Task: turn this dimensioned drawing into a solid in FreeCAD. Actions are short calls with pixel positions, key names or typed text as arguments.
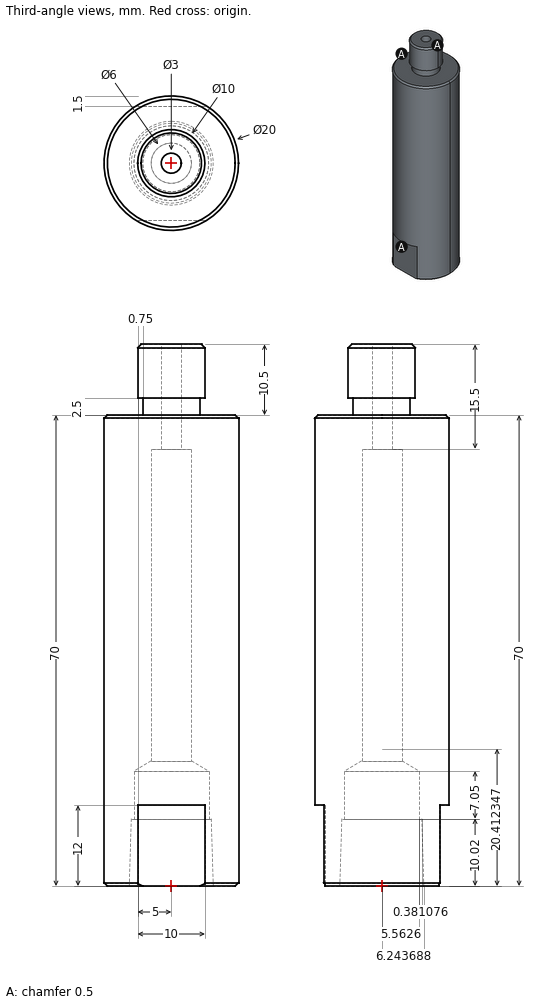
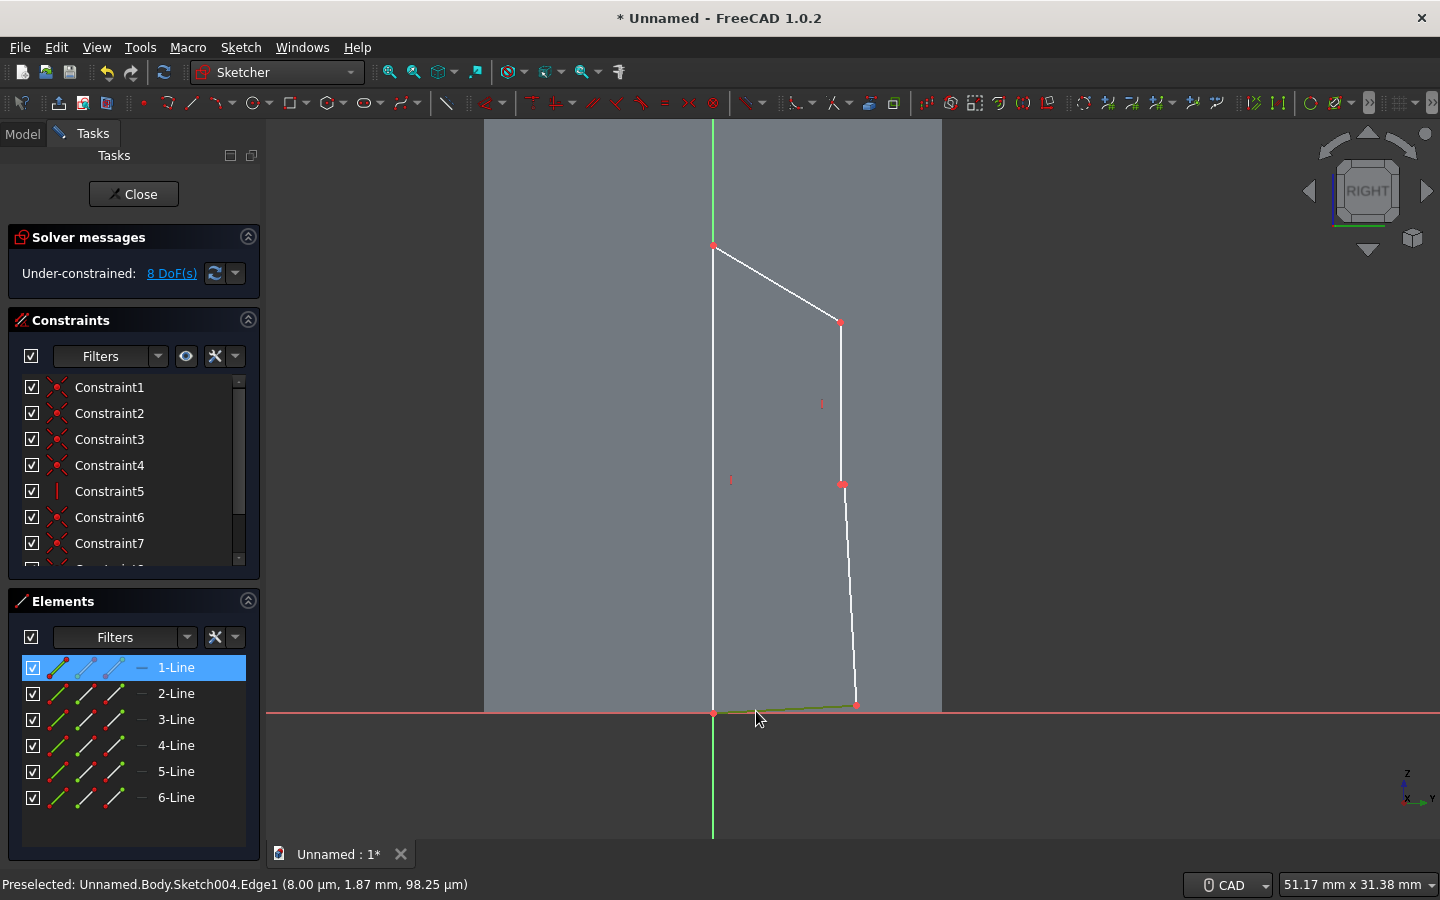
click(574, 104)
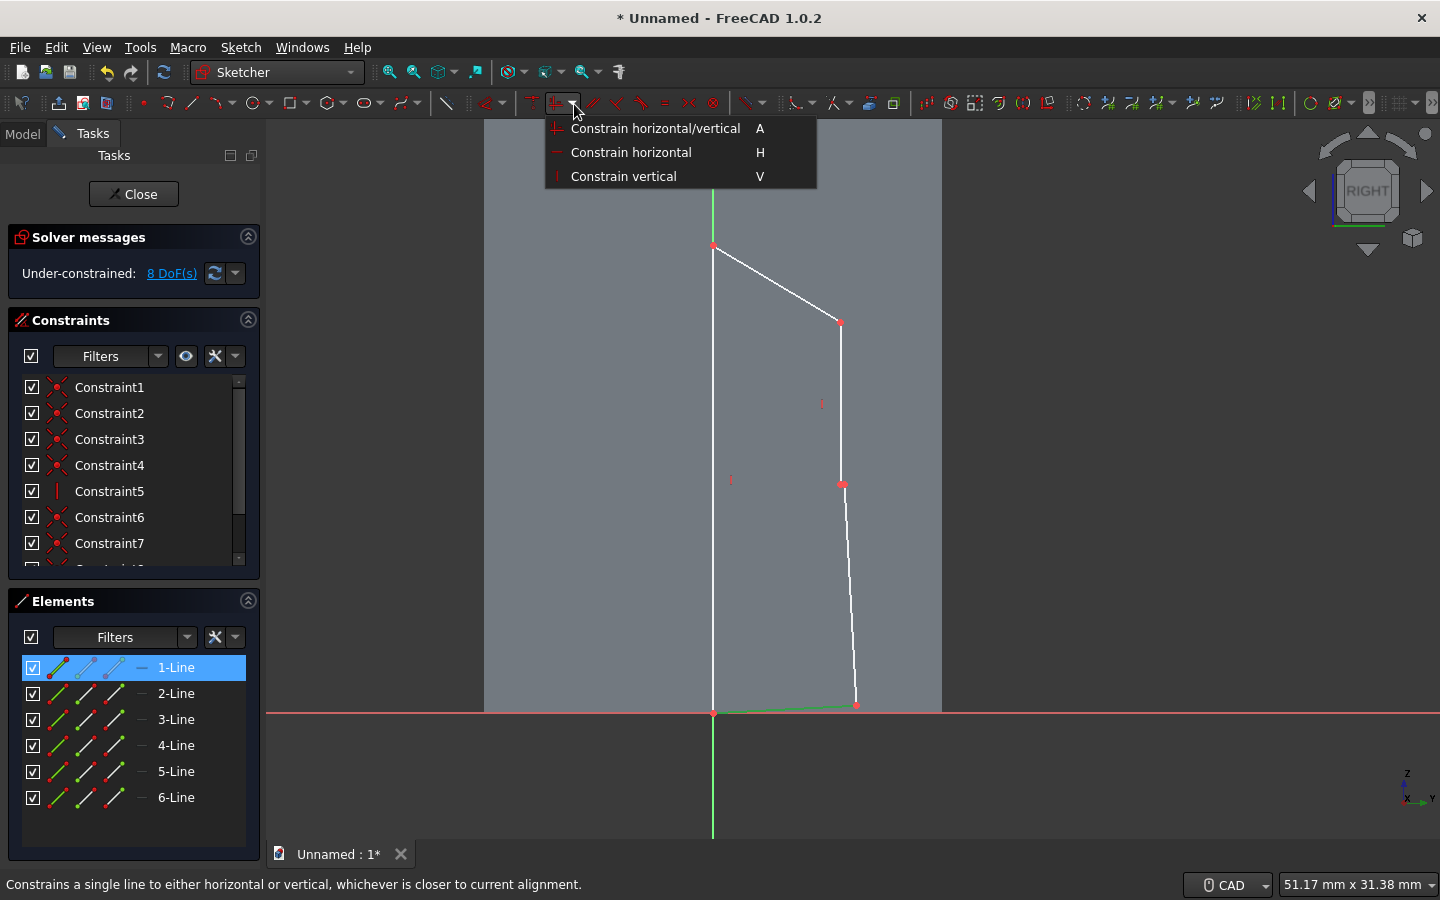
click(681, 152)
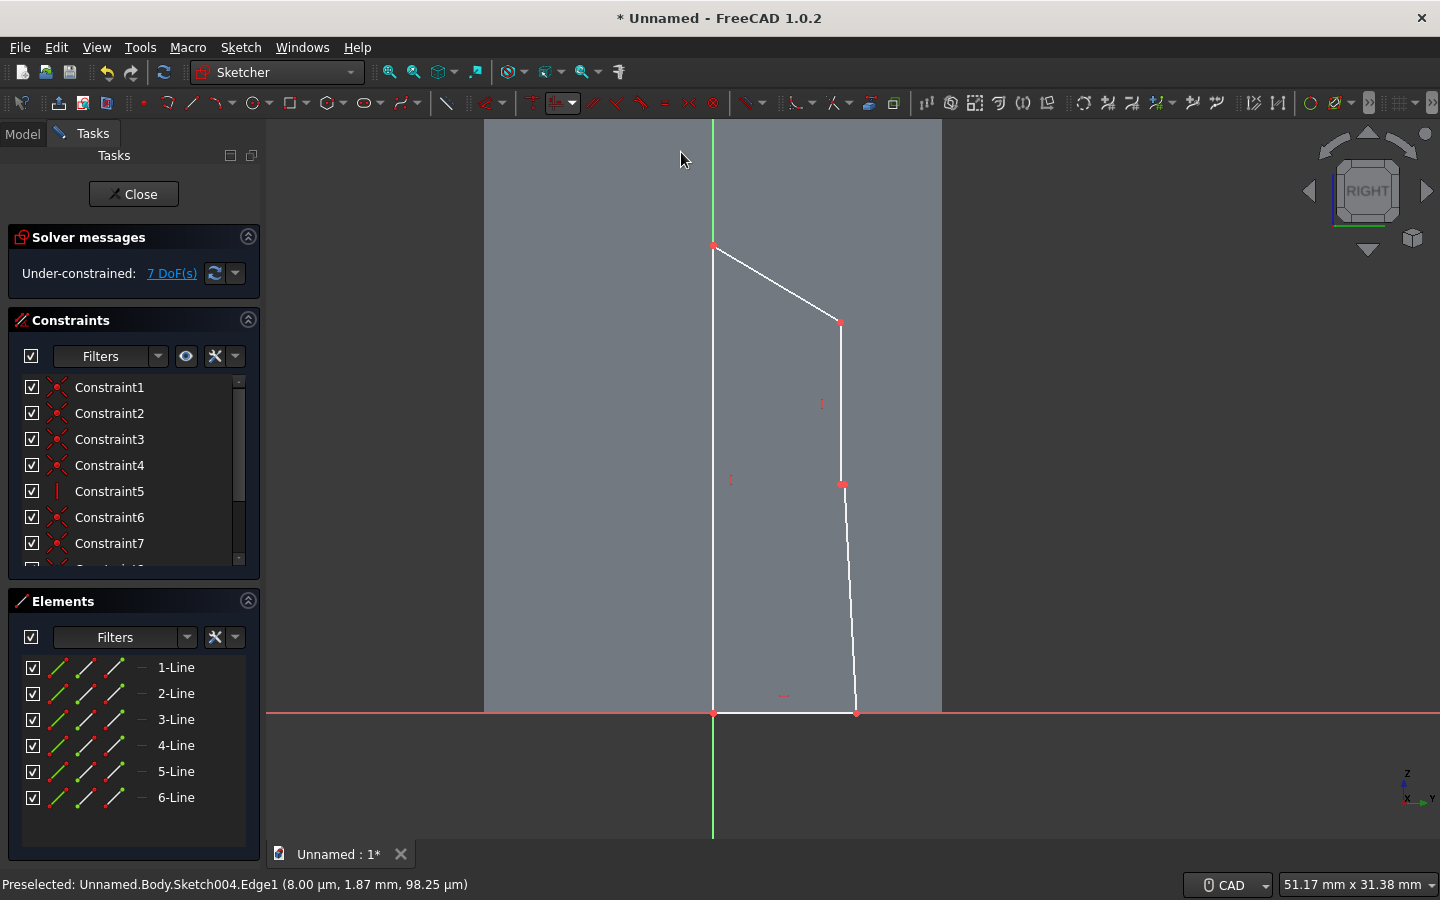
scroll(843, 485, up, 10)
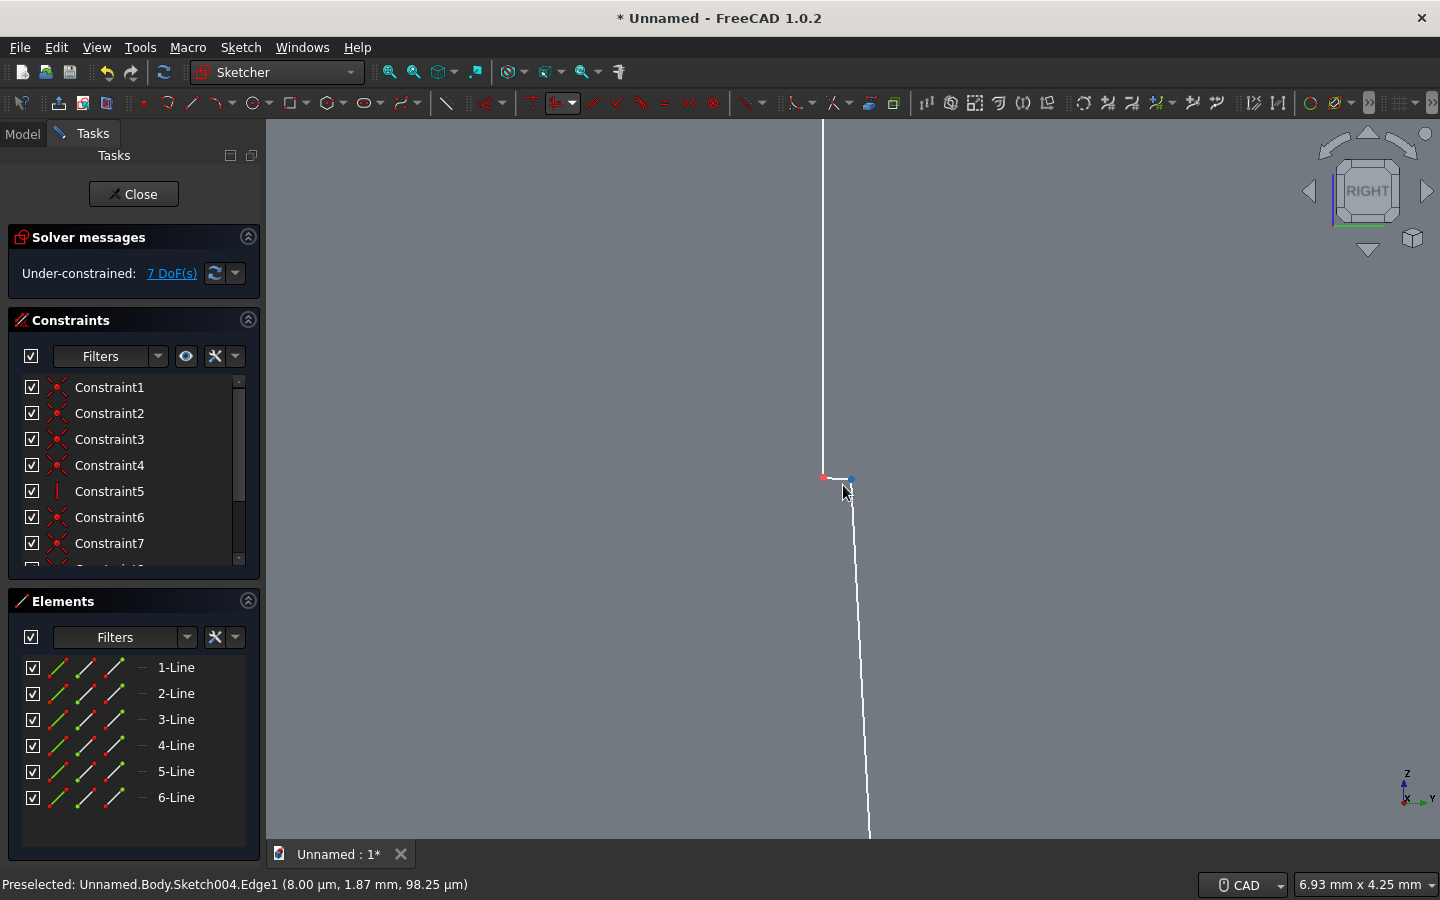
click(837, 479)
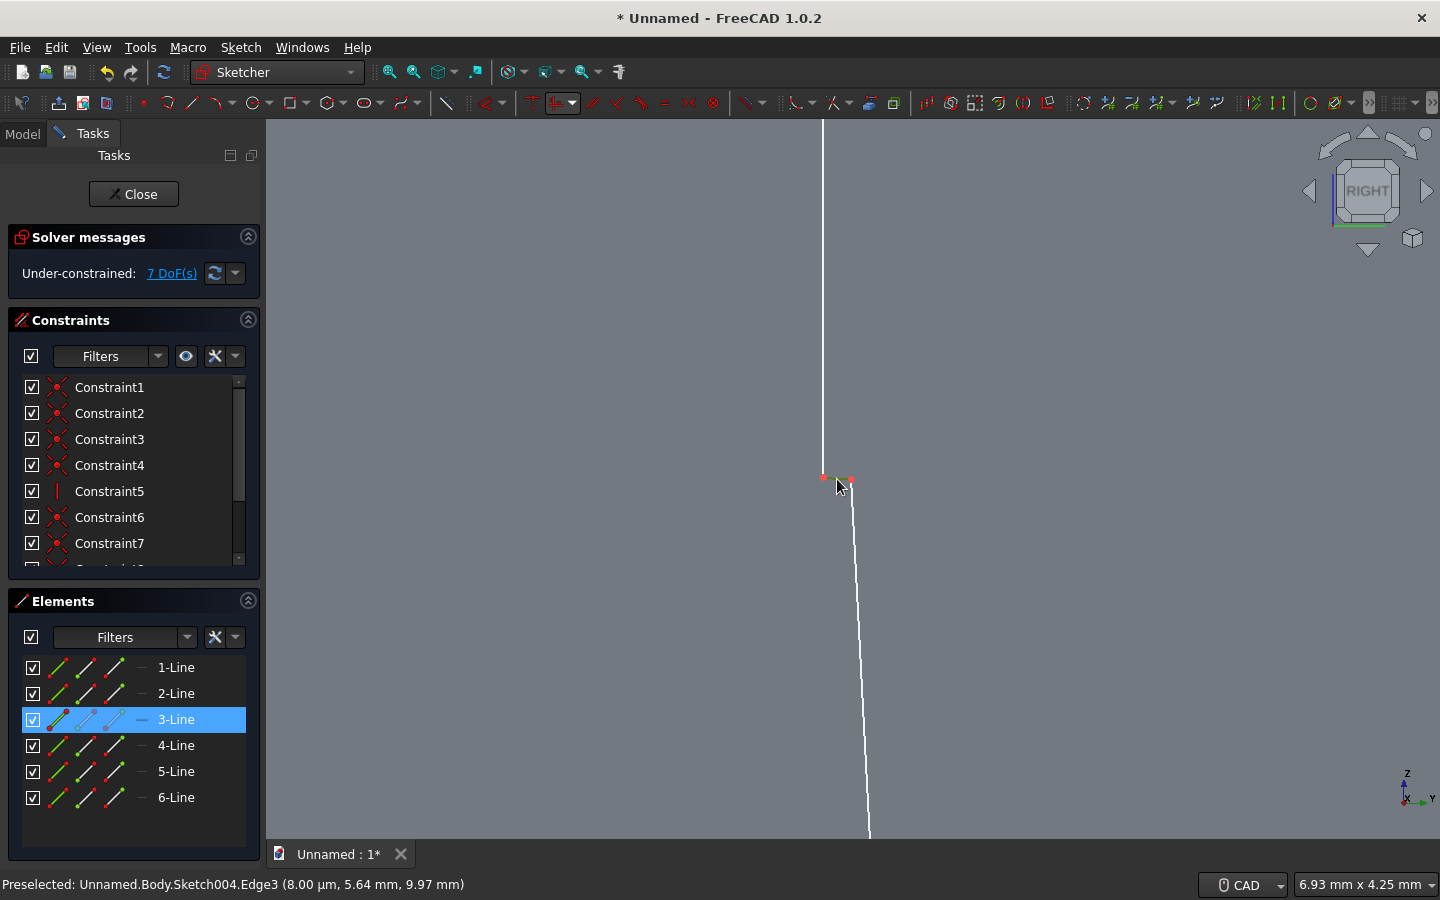
key(h)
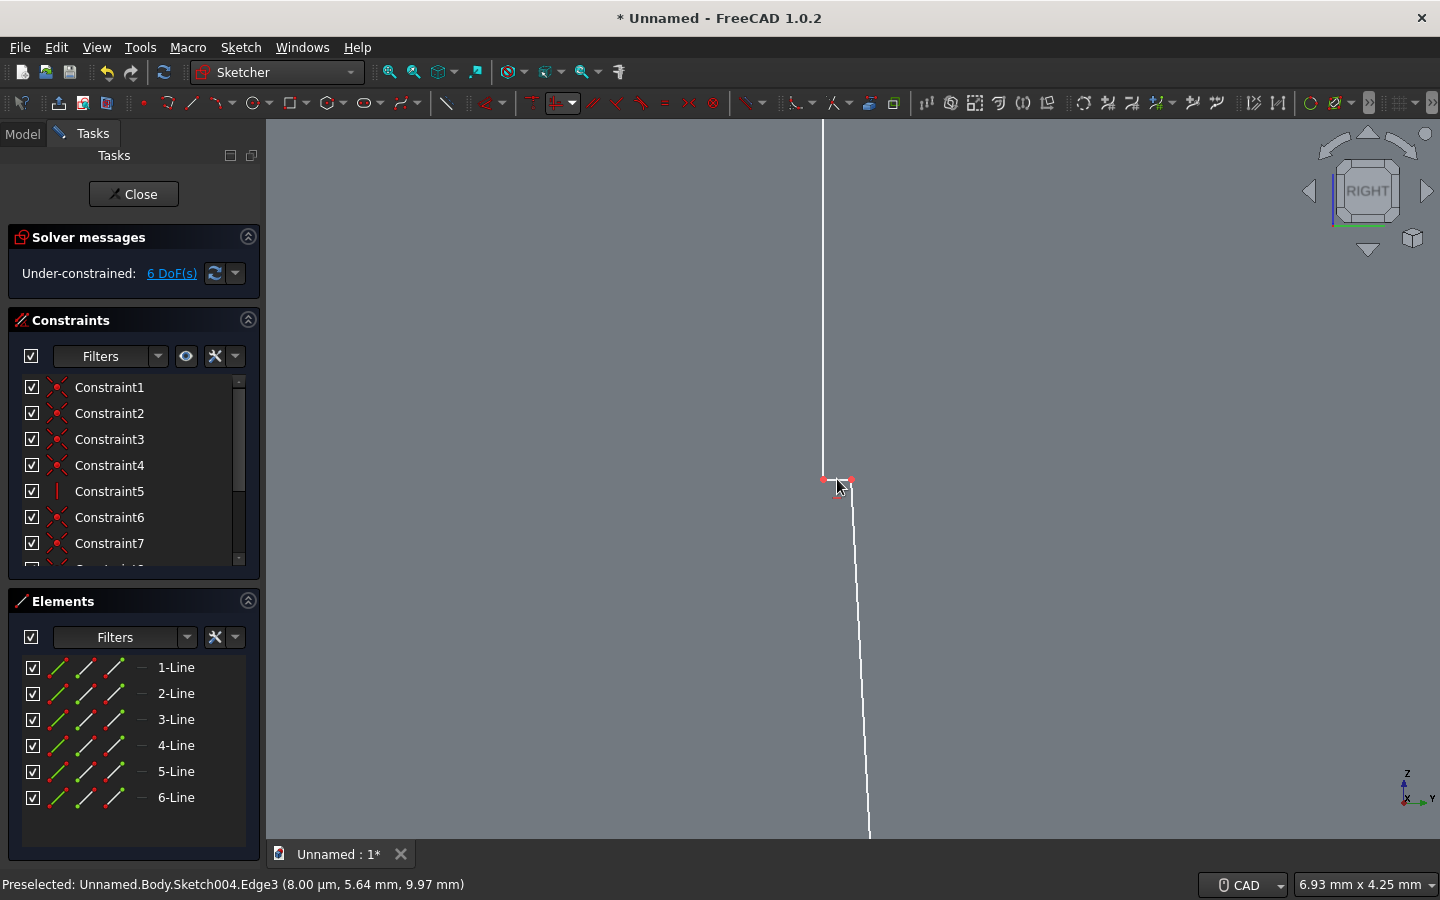
click(486, 104)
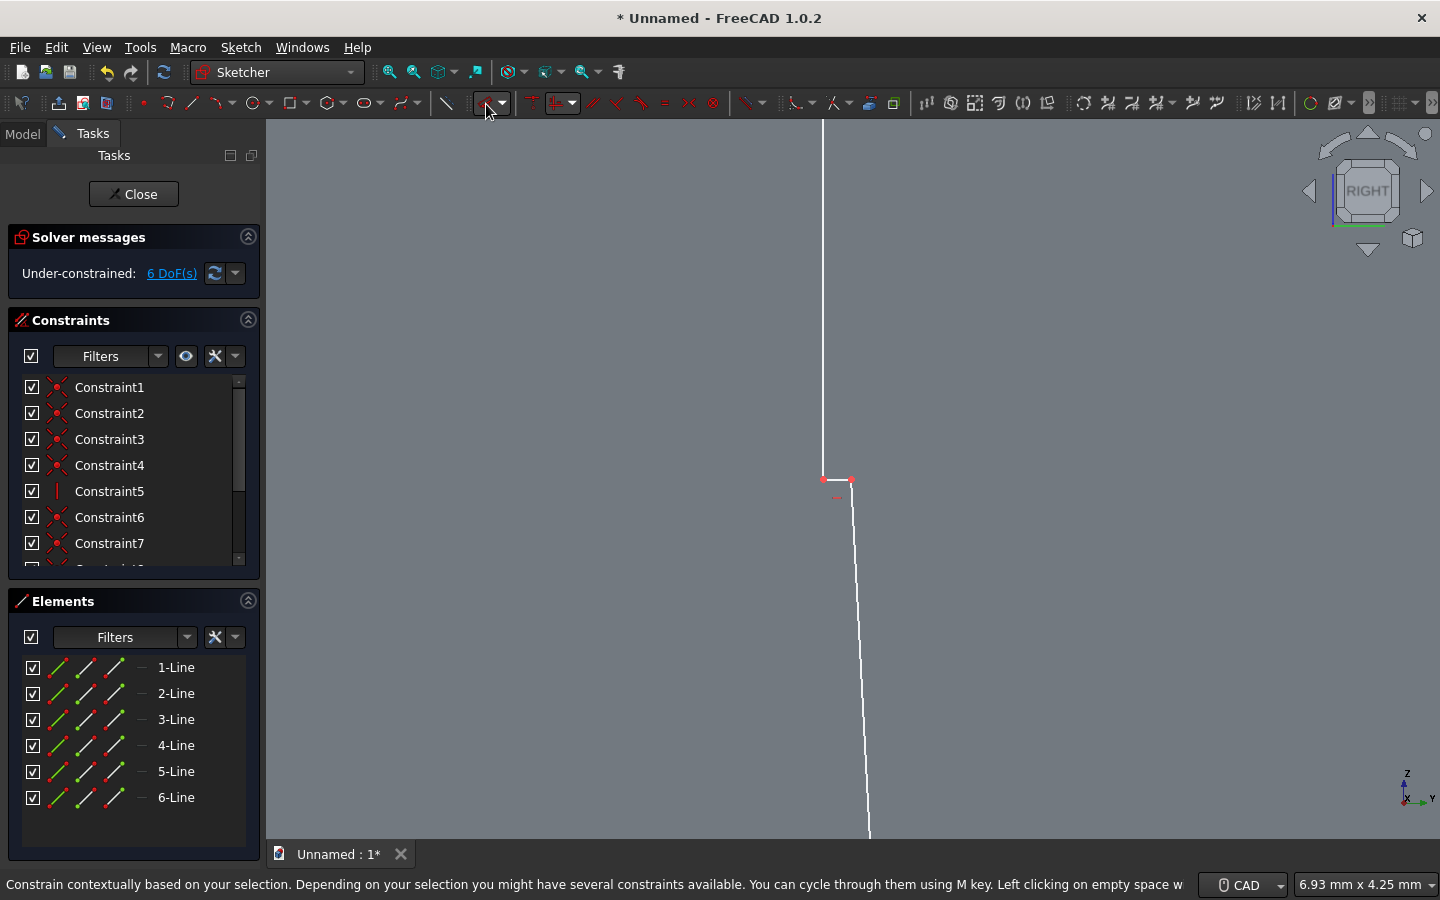
scroll(843, 485, down, 10)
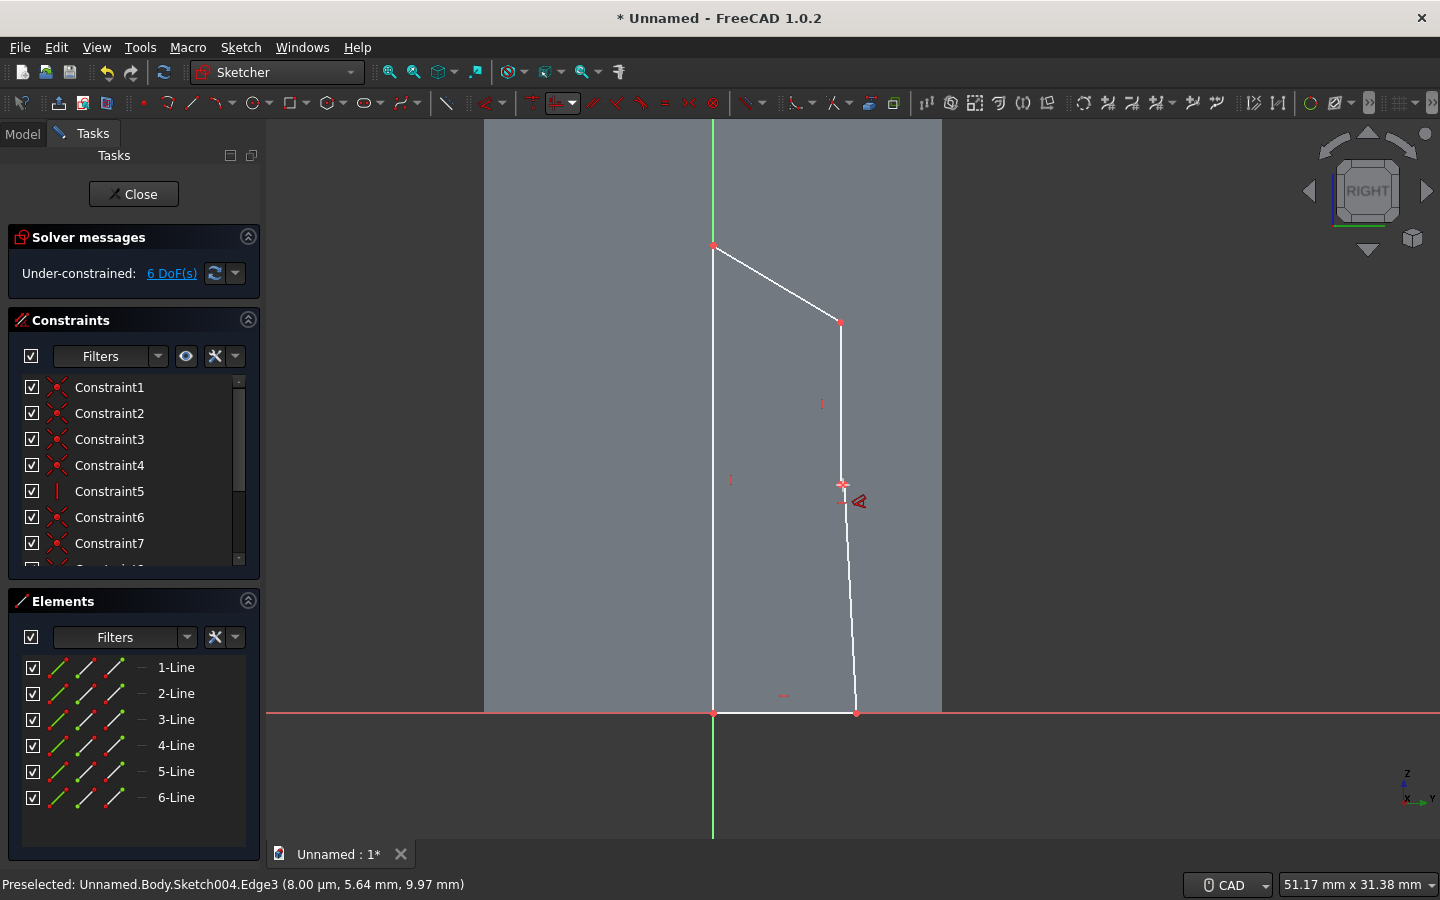
click(841, 452)
click(875, 403)